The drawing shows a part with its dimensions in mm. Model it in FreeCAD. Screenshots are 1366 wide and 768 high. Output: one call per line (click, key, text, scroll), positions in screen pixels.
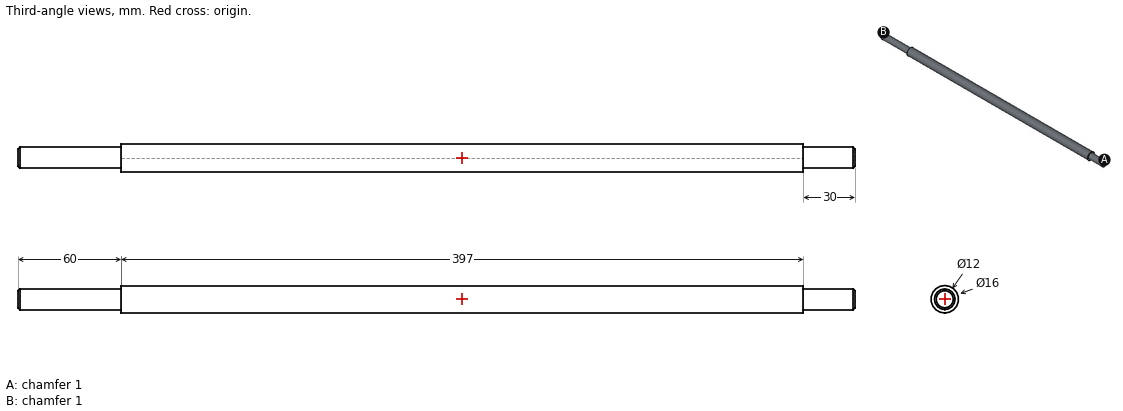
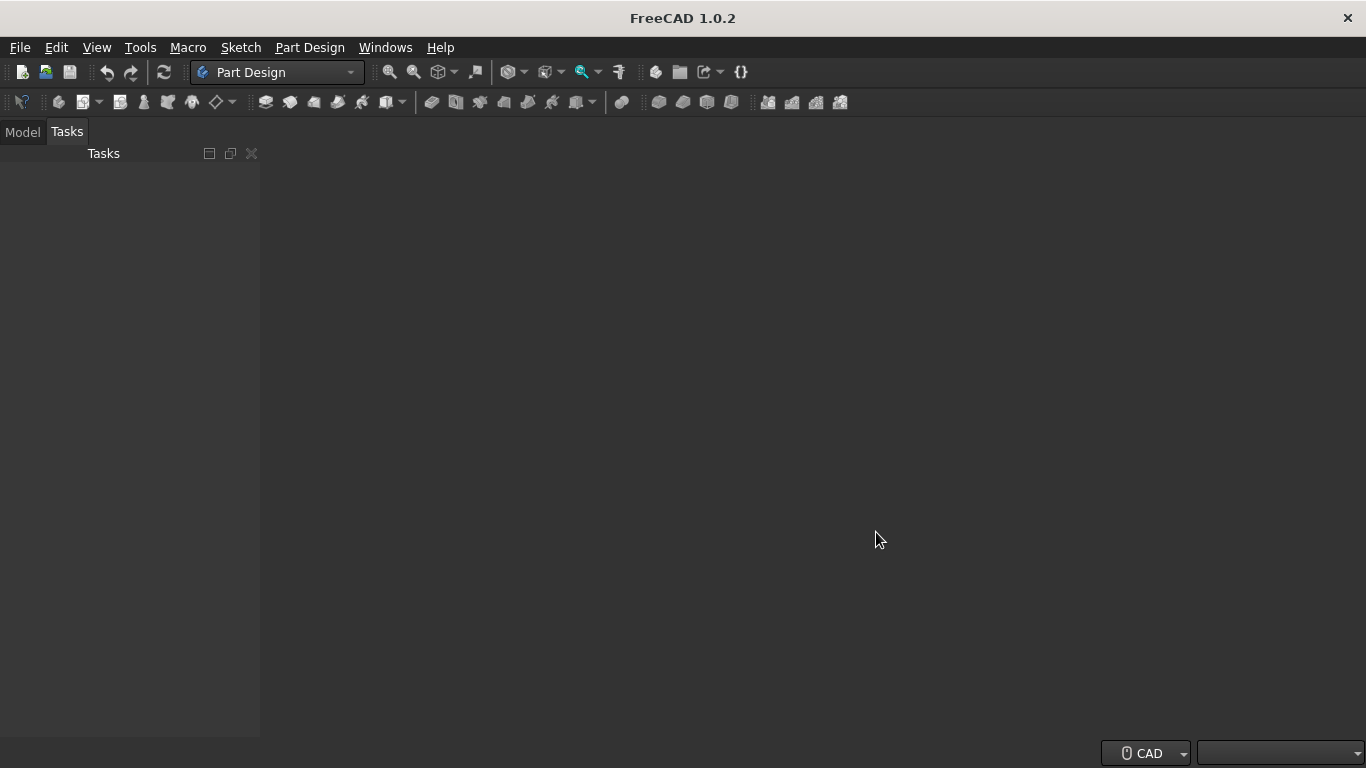
click(22, 72)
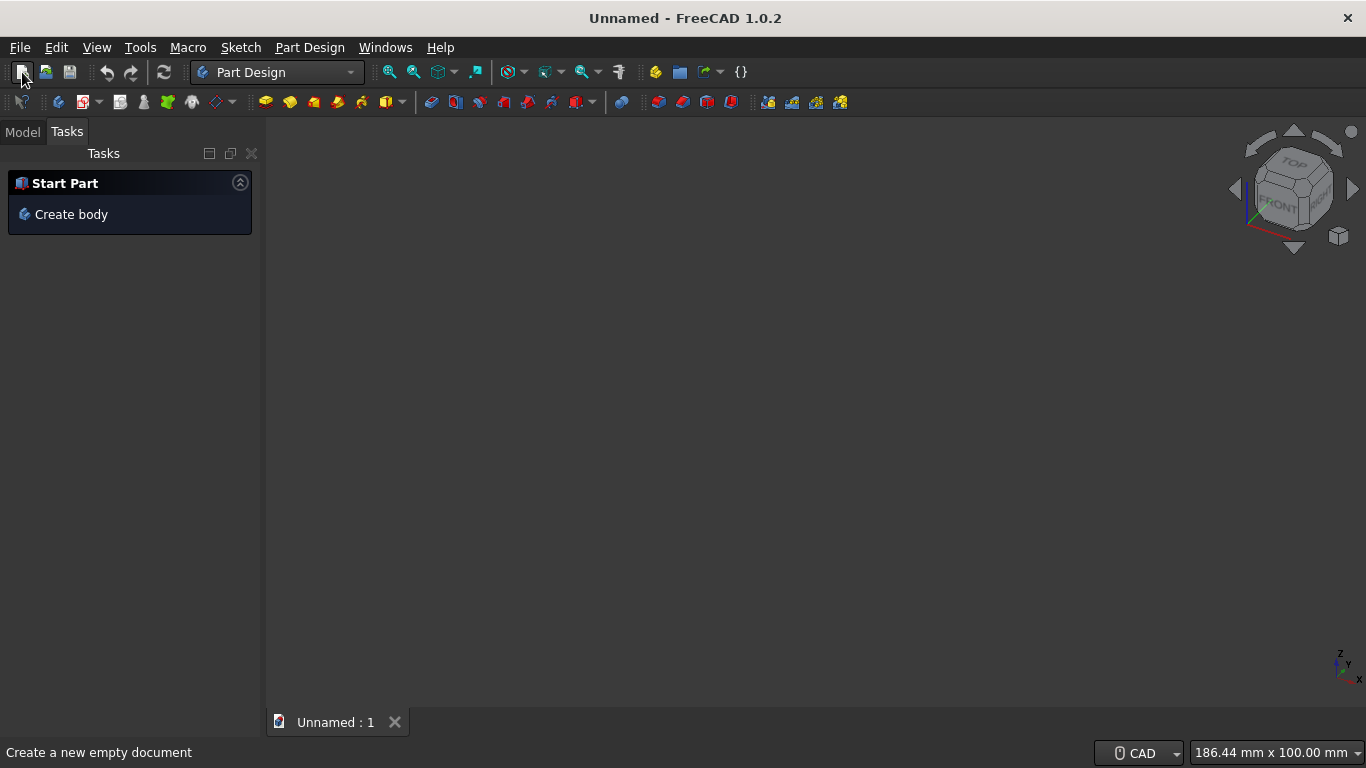
click(84, 102)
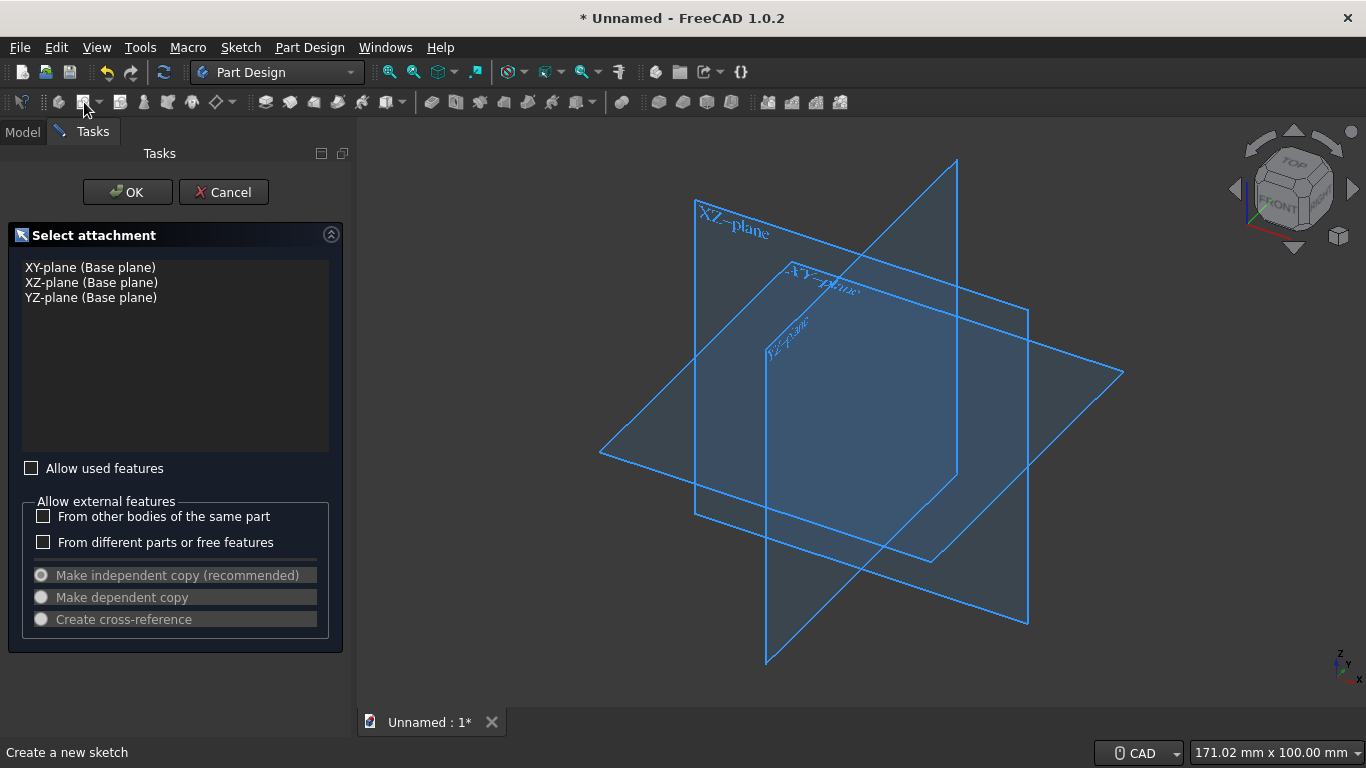
click(82, 298)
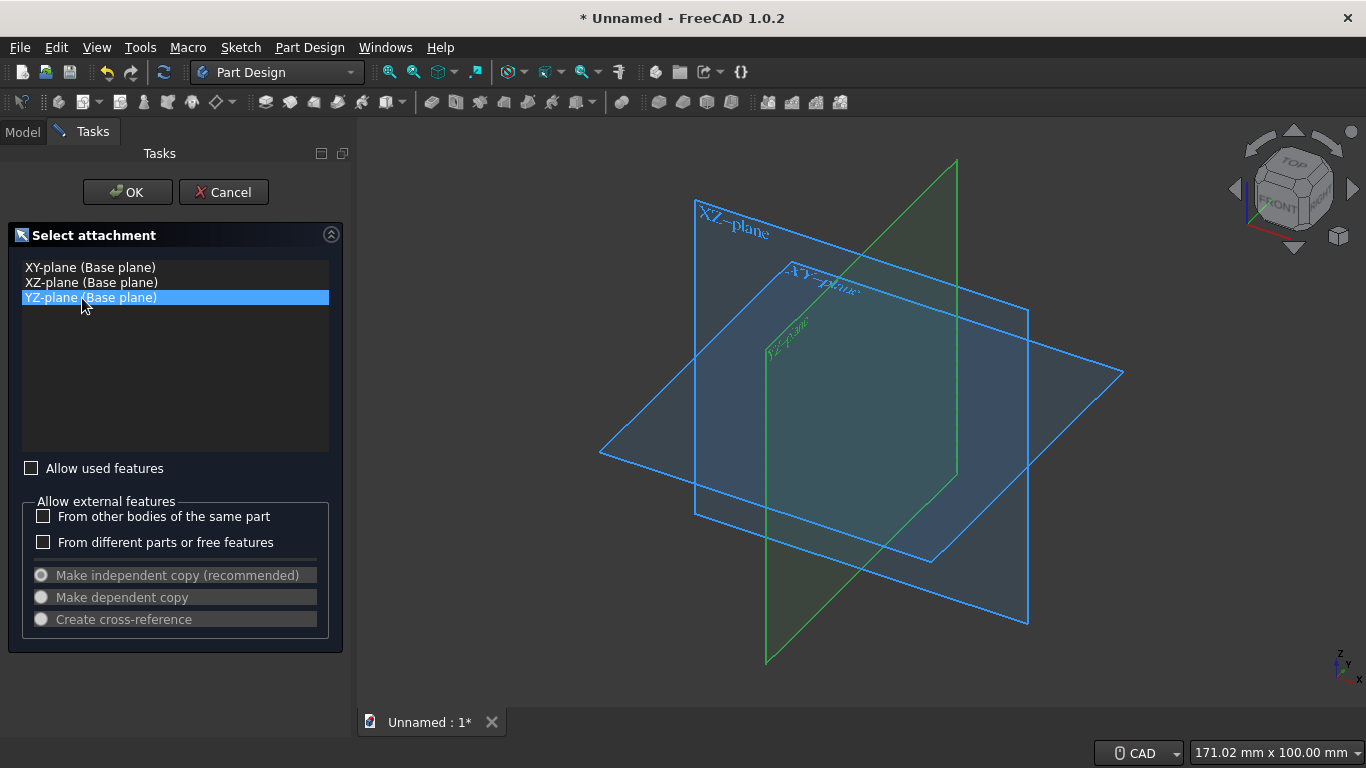
click(128, 192)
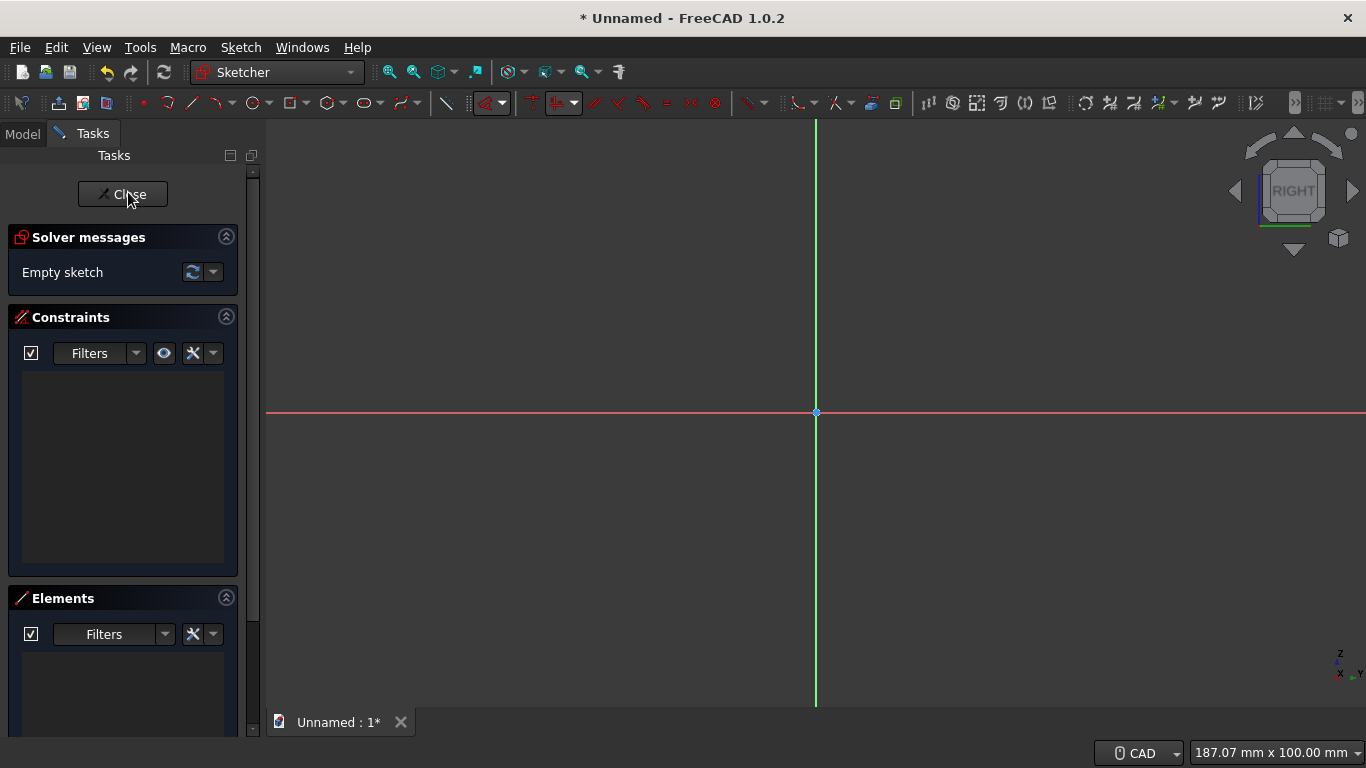
scroll(838, 413, up, 7)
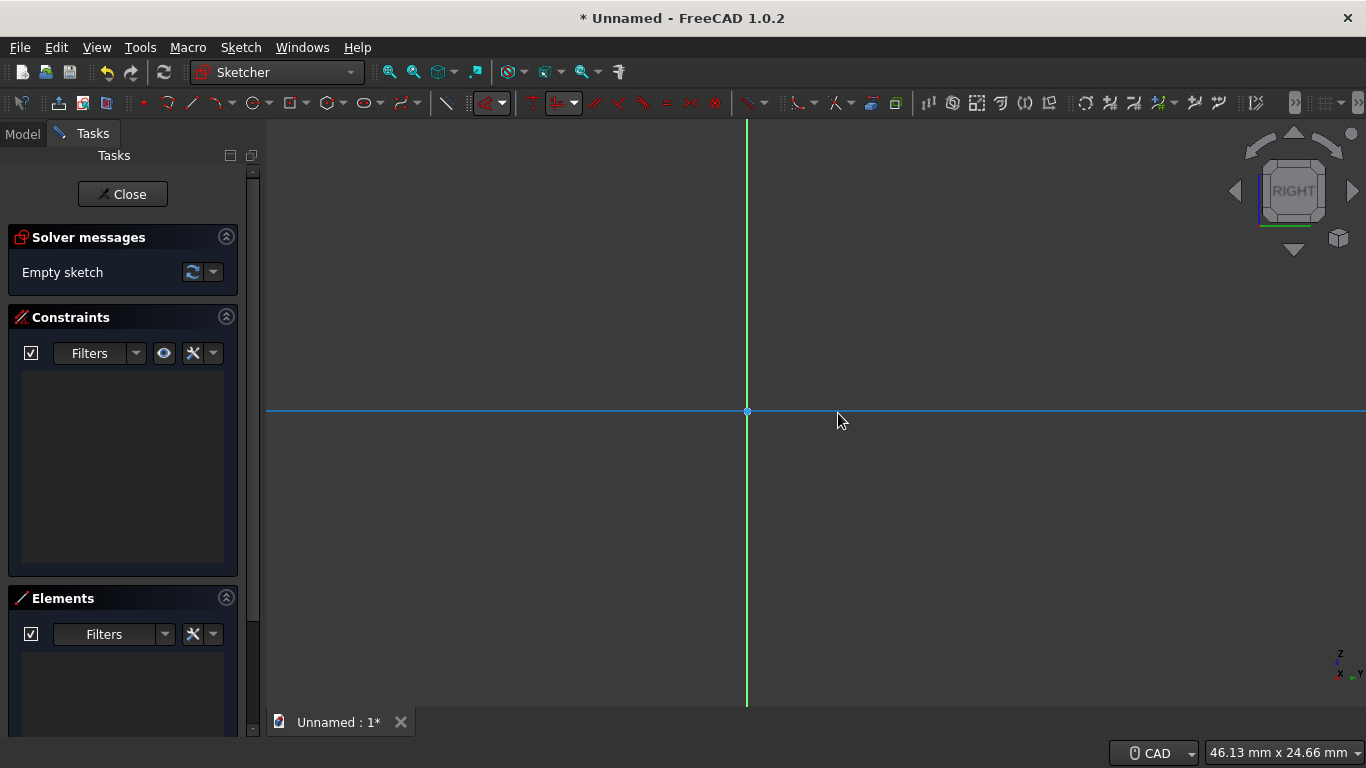
click(254, 104)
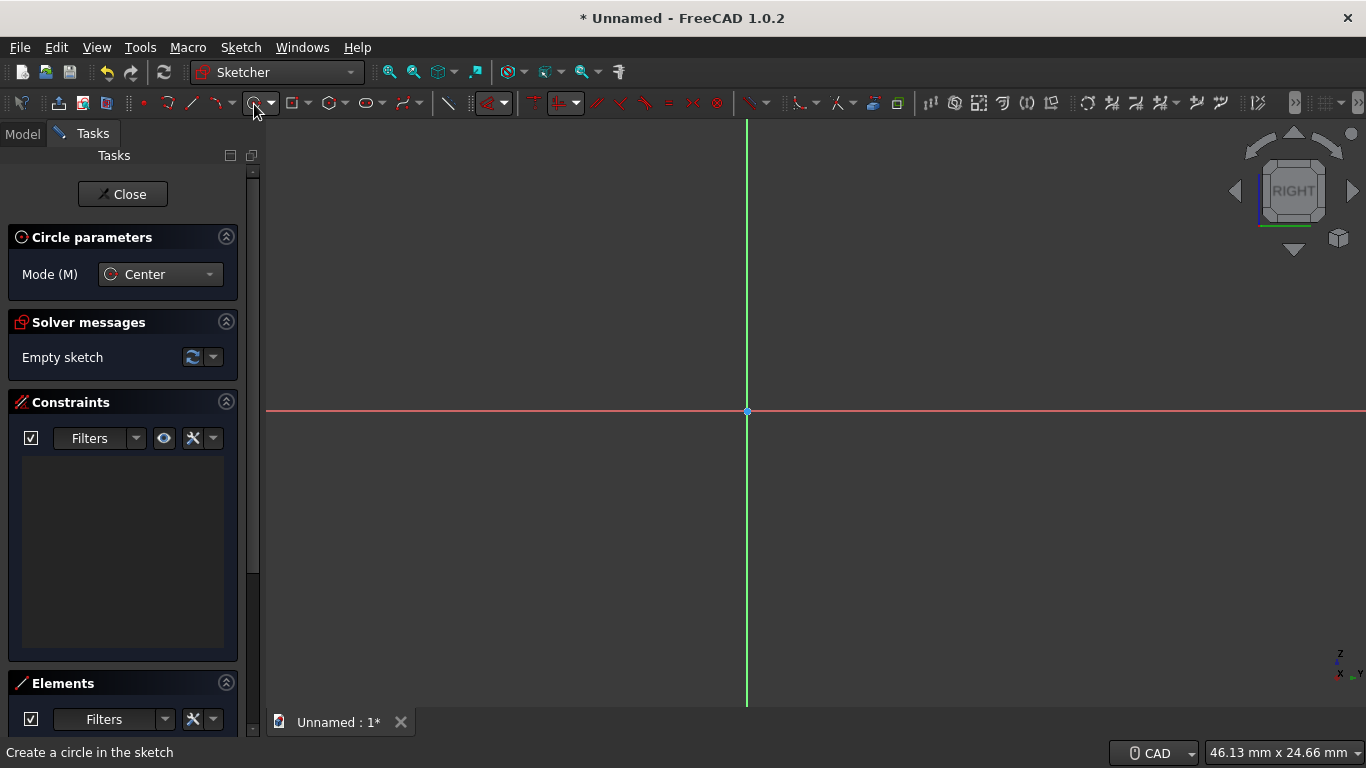
click(747, 411)
move(882, 277)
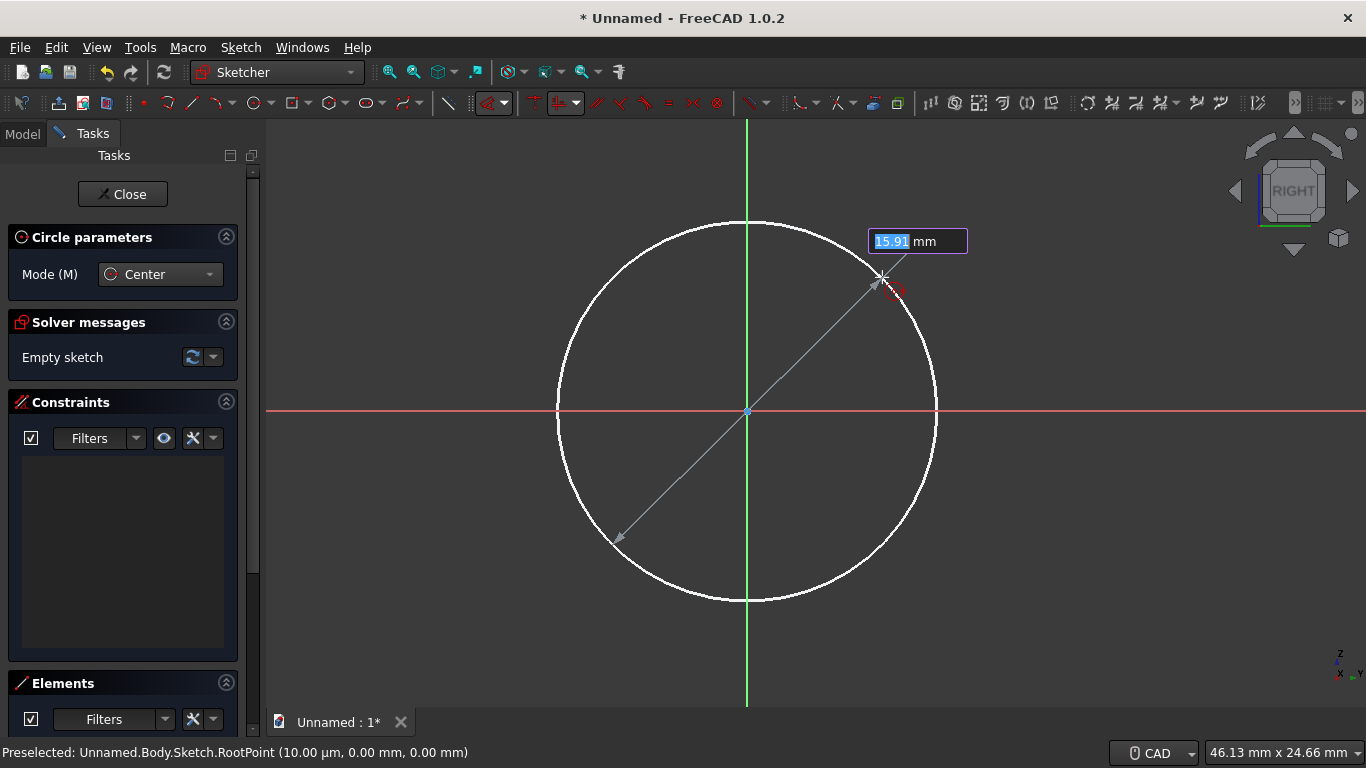
text(16)
key(Return)
key(Escape)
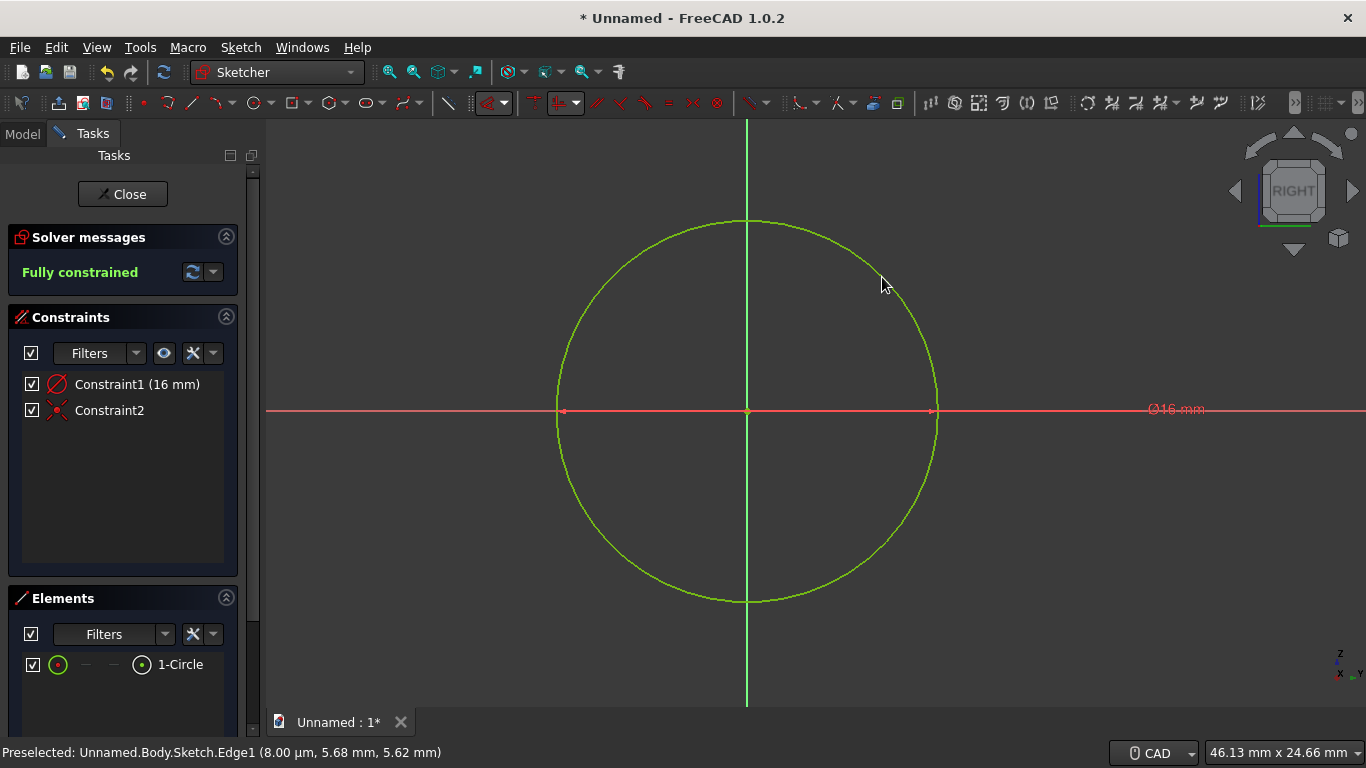
click(123, 194)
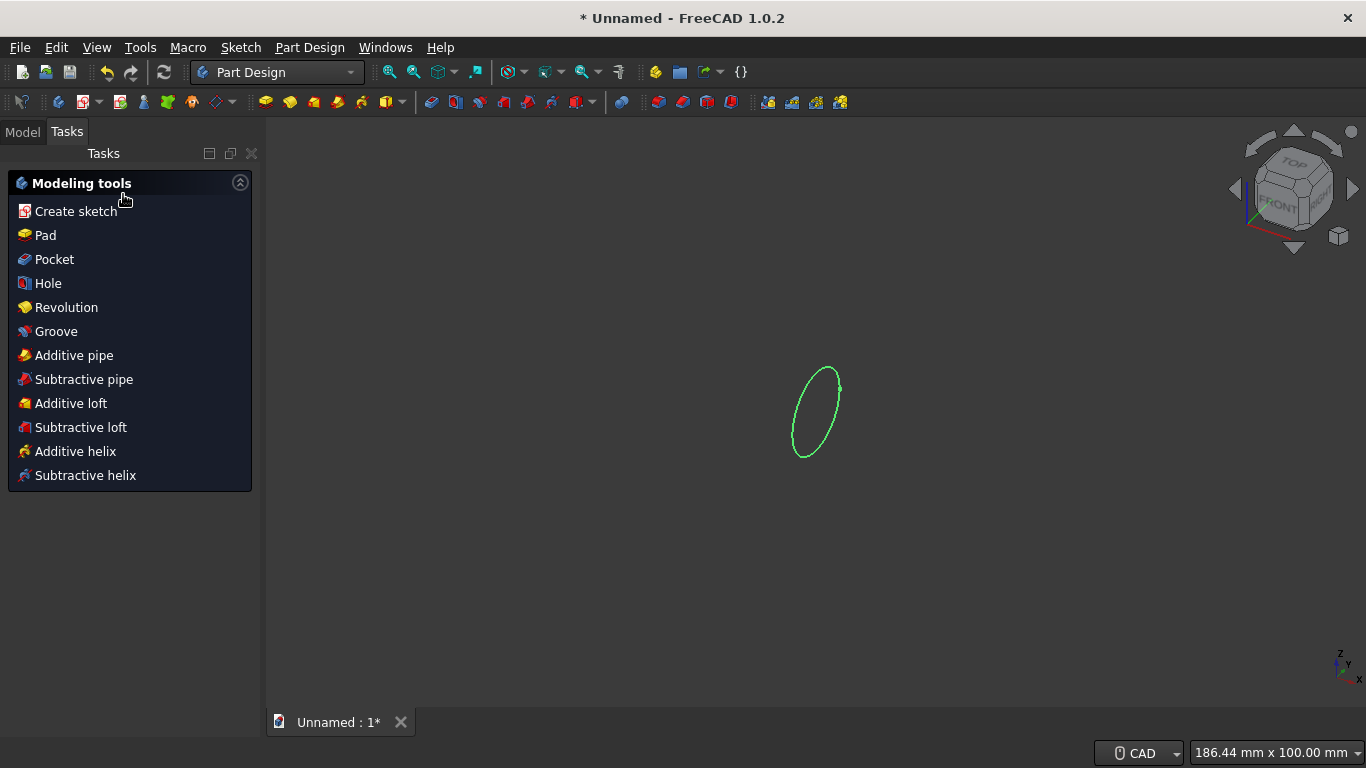
click(266, 102)